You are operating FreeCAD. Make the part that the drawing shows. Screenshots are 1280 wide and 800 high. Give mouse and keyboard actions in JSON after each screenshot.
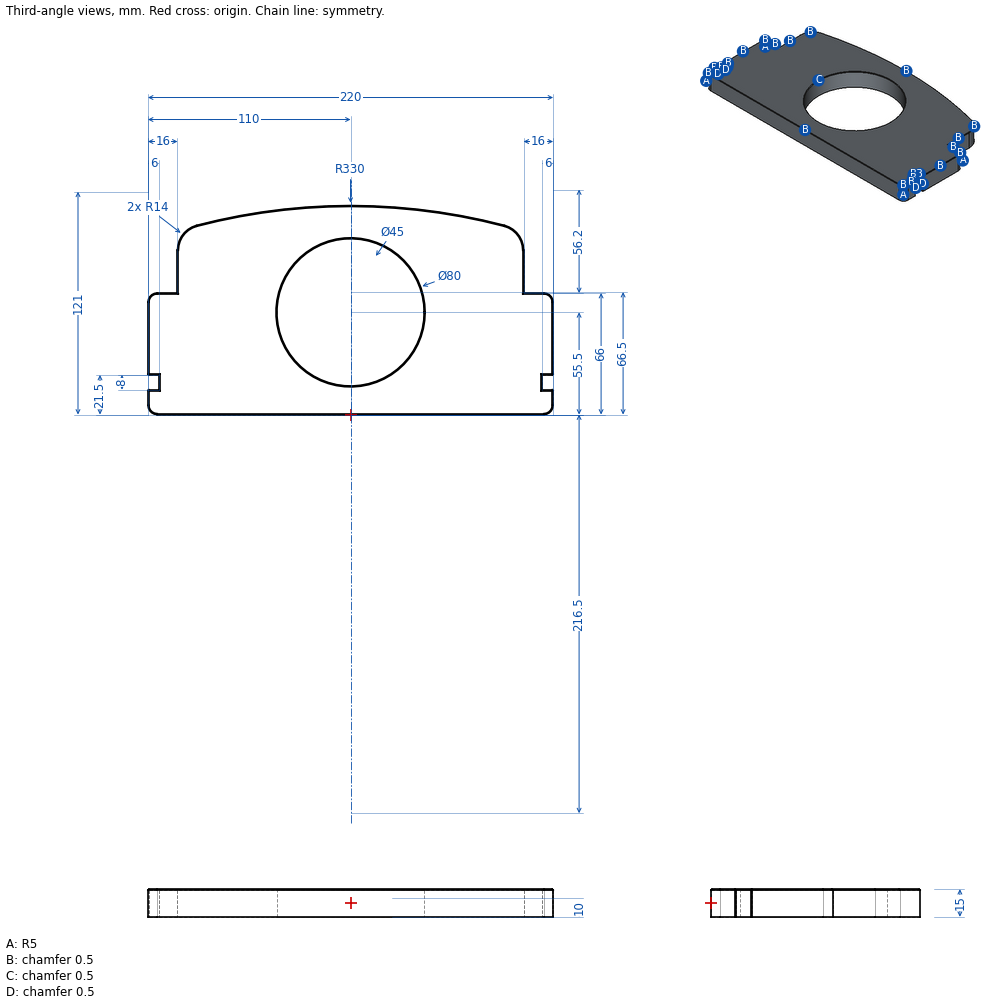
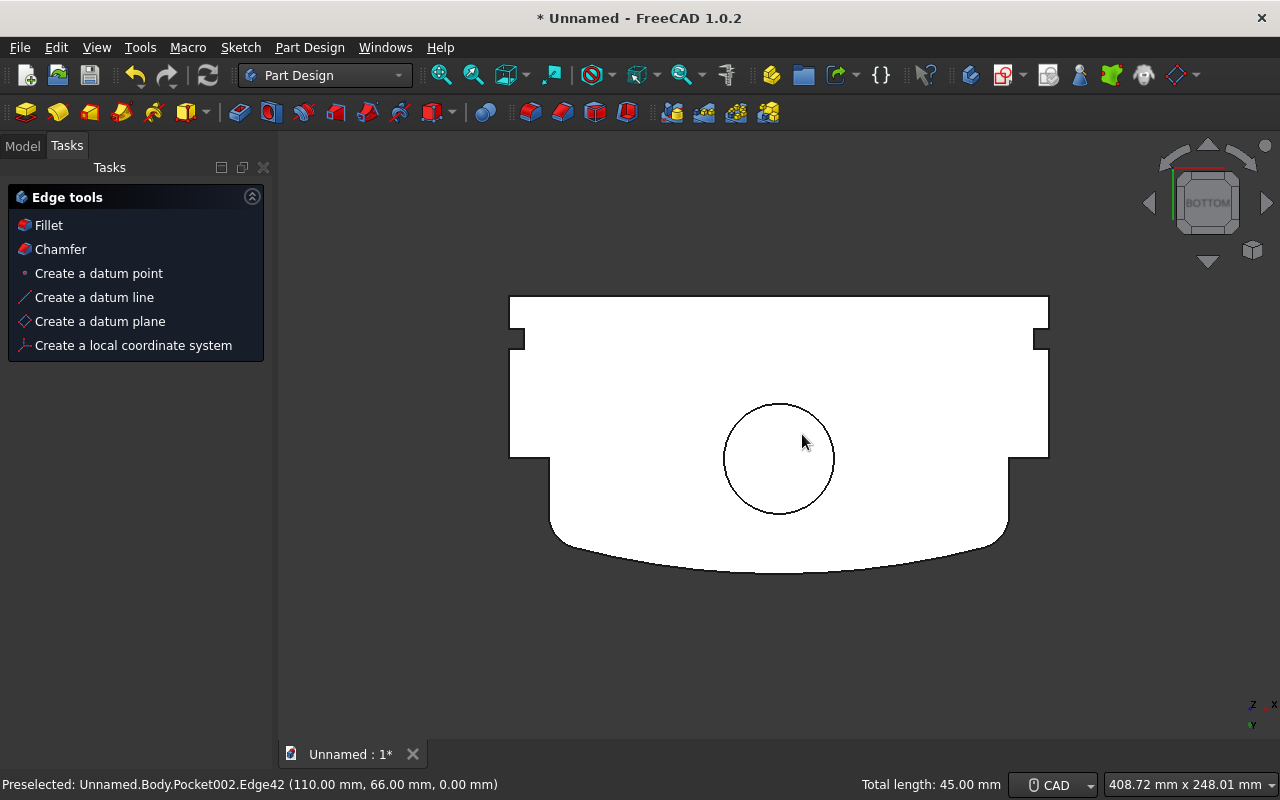
{"action": "key", "text": "4"}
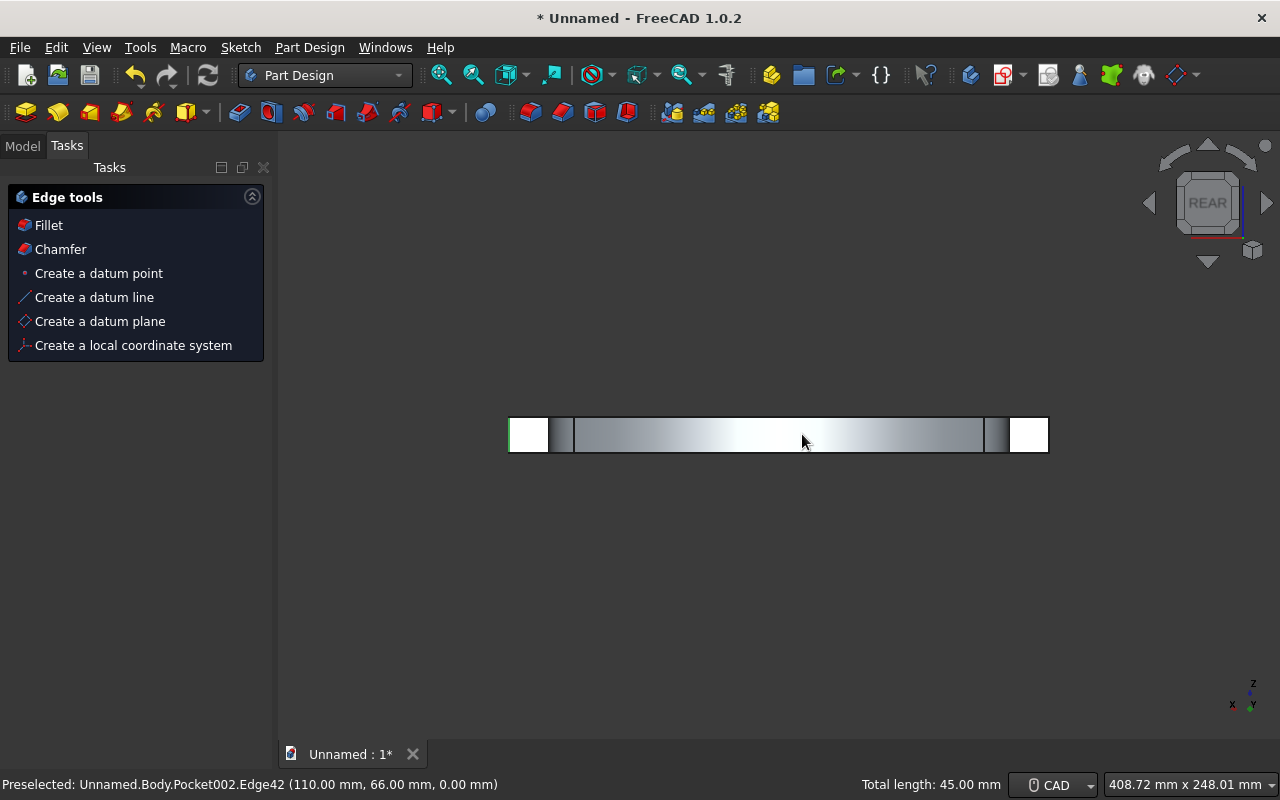
{"action": "left_click", "coordinate": [1049, 434], "text": "ctrl"}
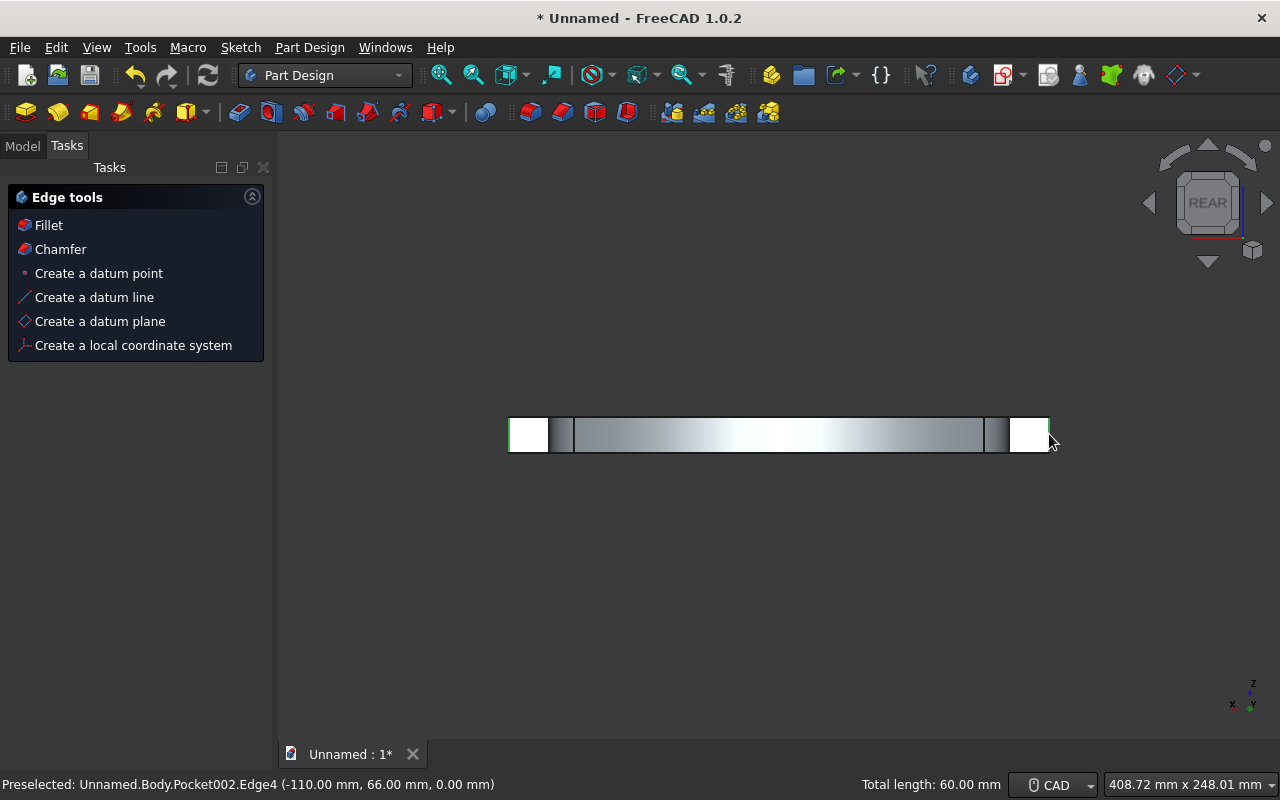
{"action": "left_click", "coordinate": [532, 112]}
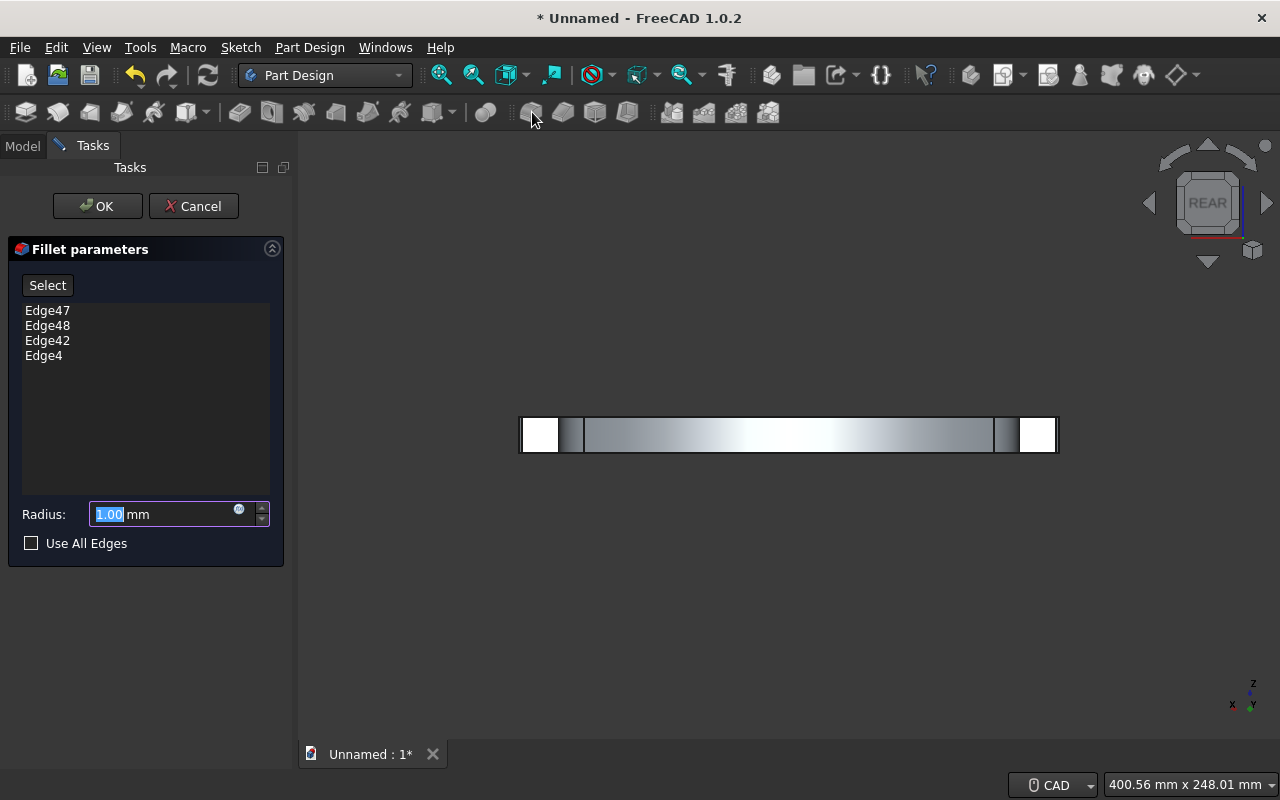
{"action": "type", "text": "5"}
{"action": "key", "text": "Tab"}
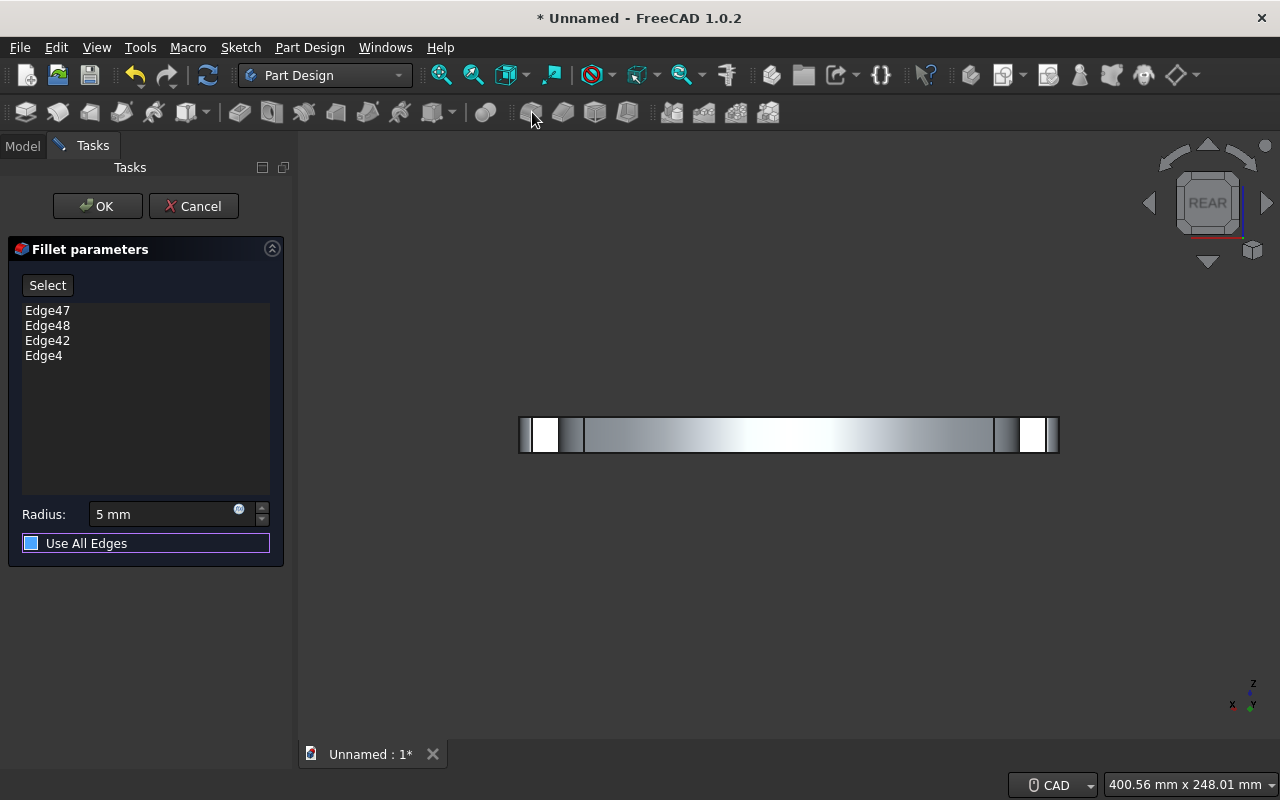
{"action": "left_click", "coordinate": [98, 206]}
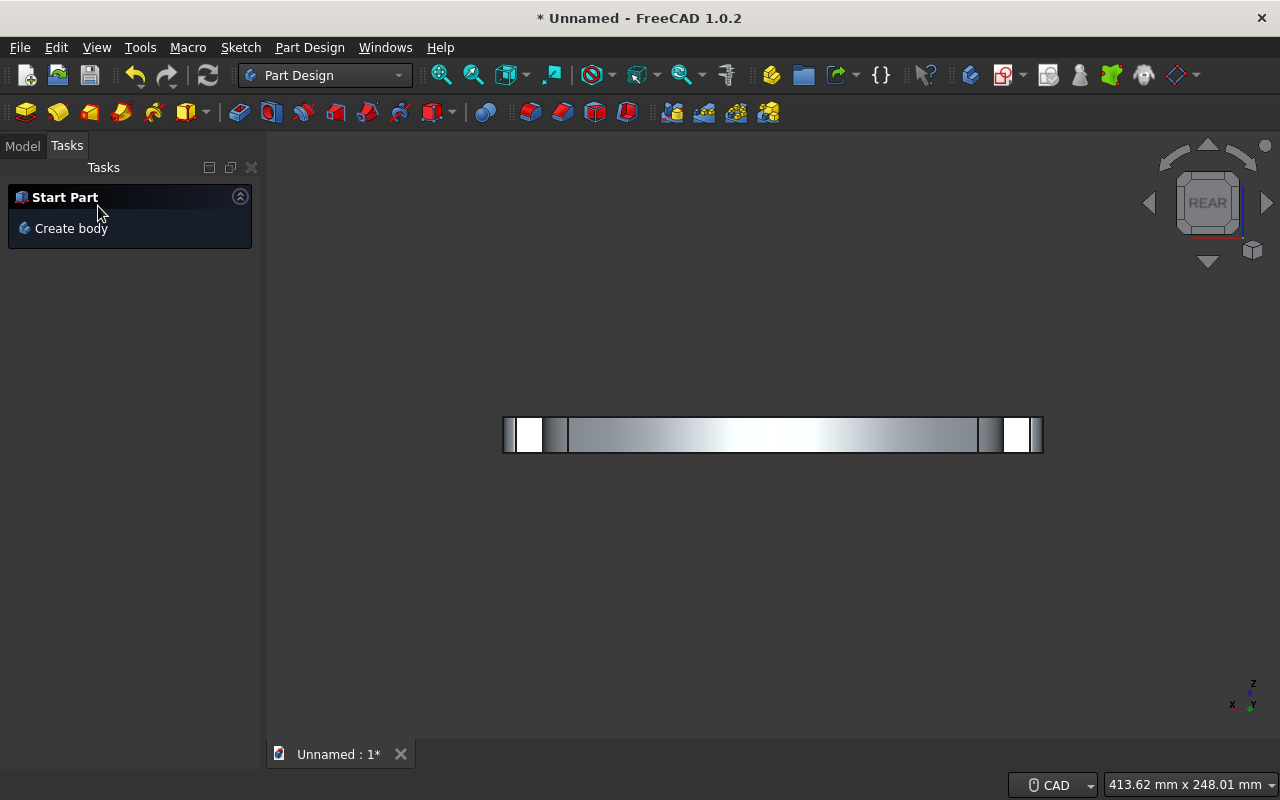
{"action": "key", "text": "0"}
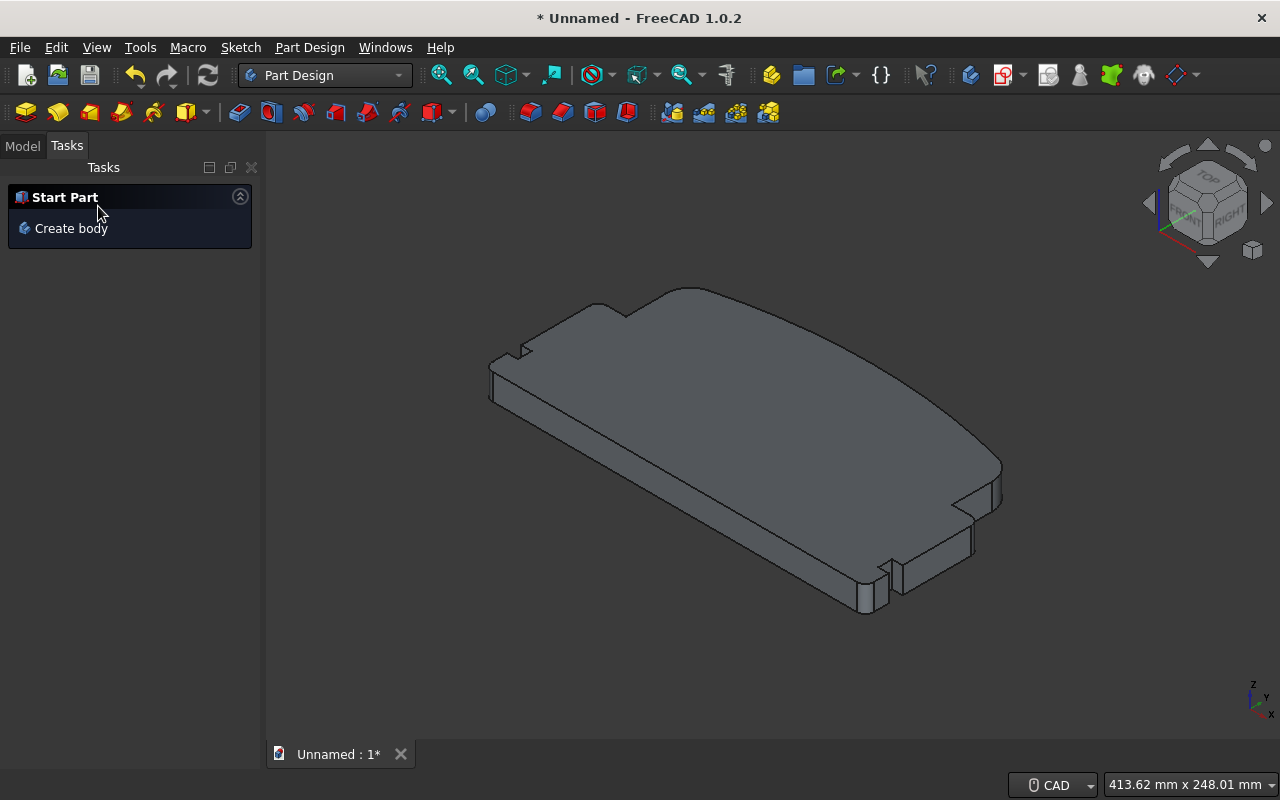
{"action": "left_click", "coordinate": [773, 419]}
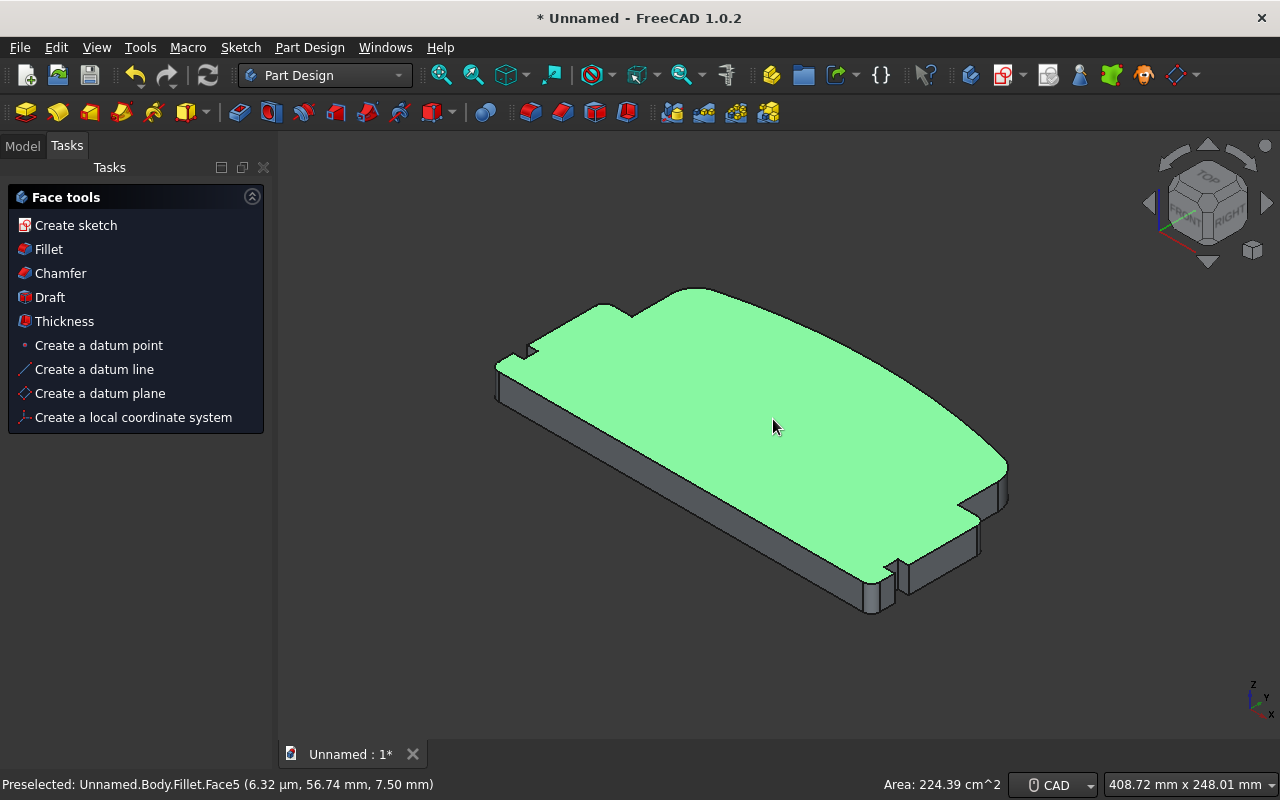
{"action": "left_click", "coordinate": [564, 112]}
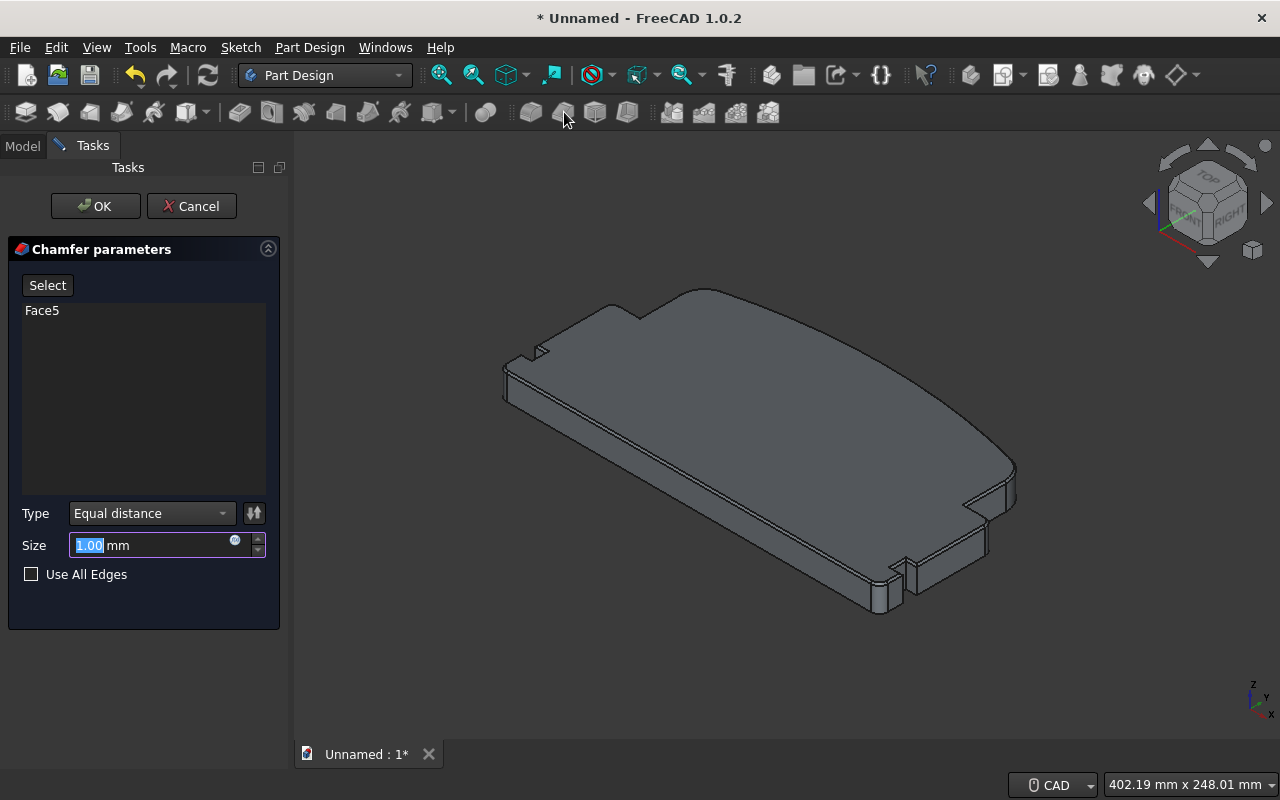
{"action": "type", "text": "0.5"}
{"action": "key", "text": "Tab"}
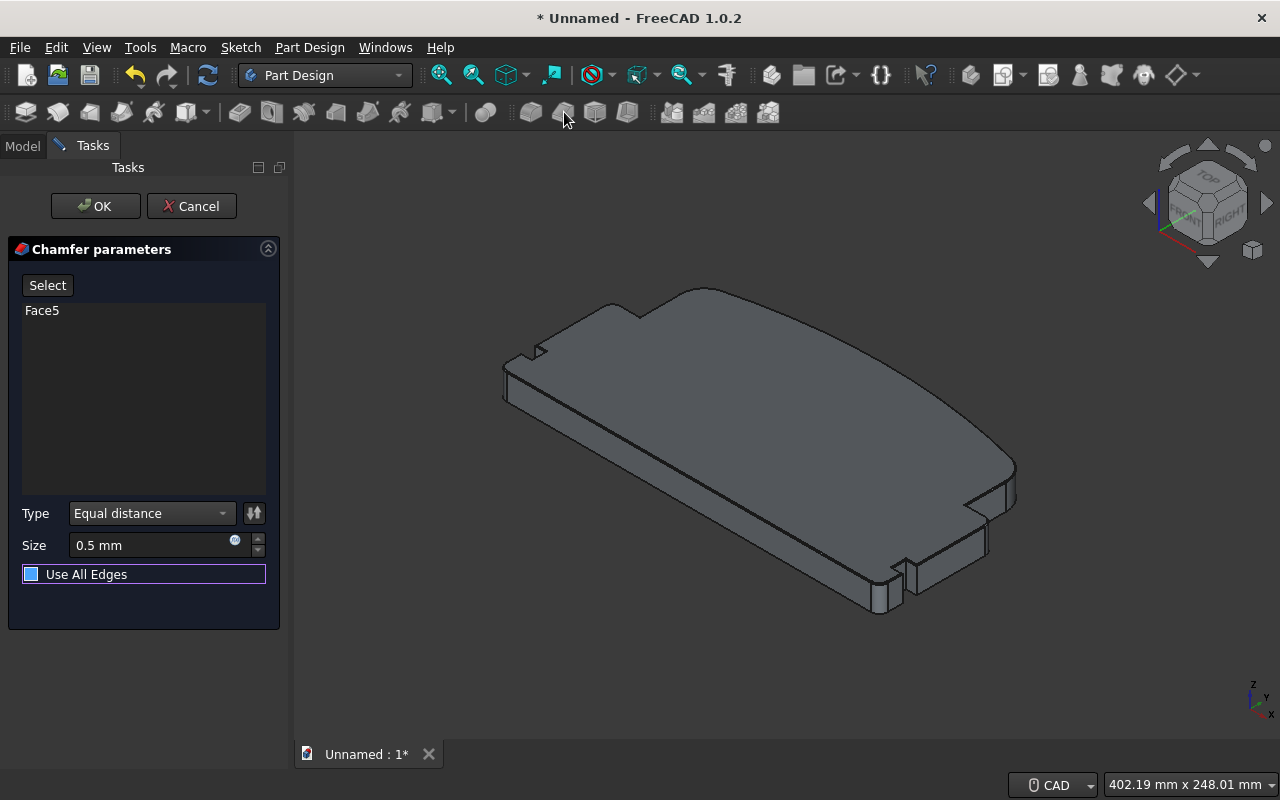
{"action": "left_click", "coordinate": [96, 206]}